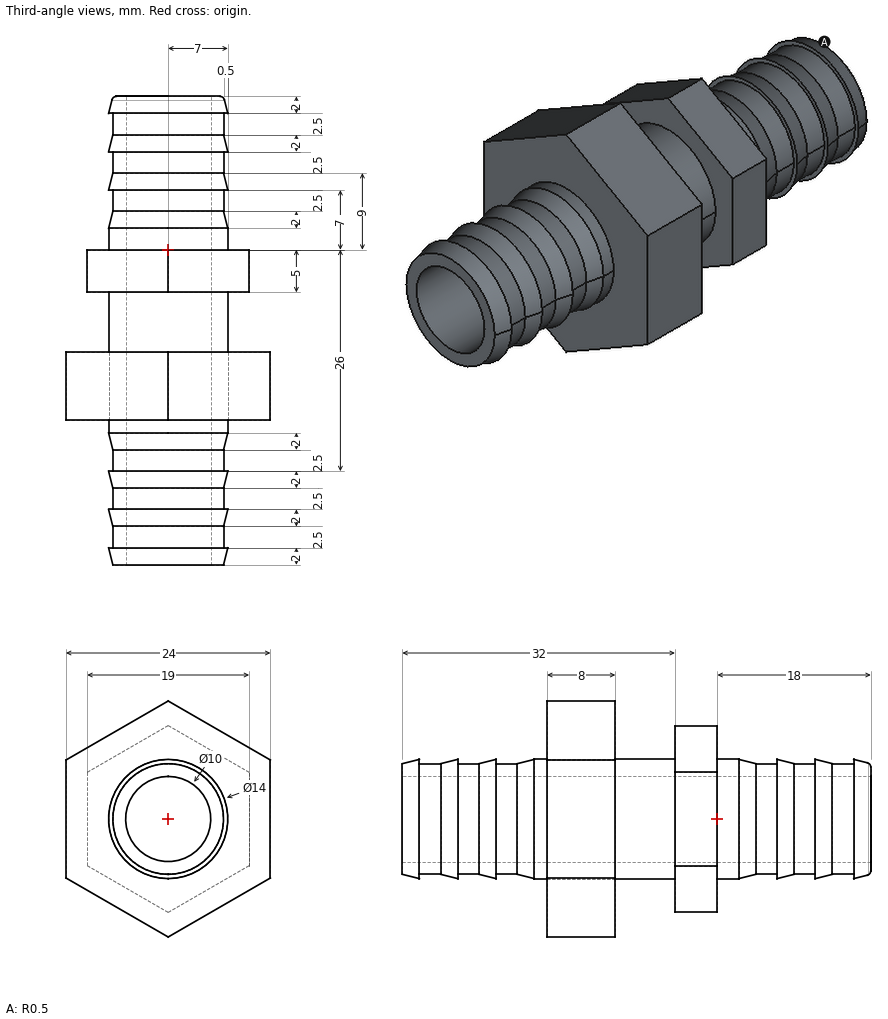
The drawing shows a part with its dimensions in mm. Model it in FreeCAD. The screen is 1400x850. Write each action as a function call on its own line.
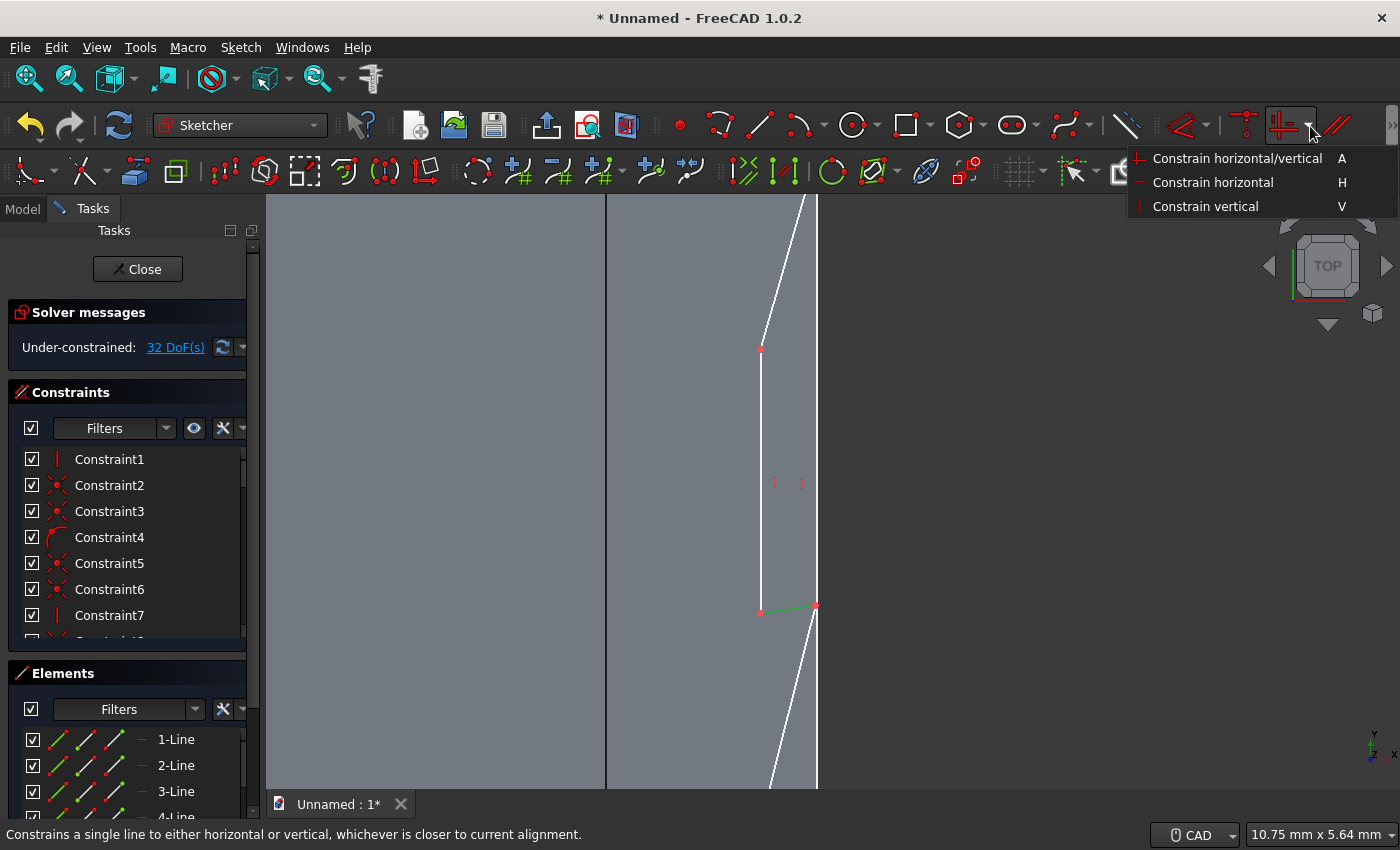
click(1263, 182)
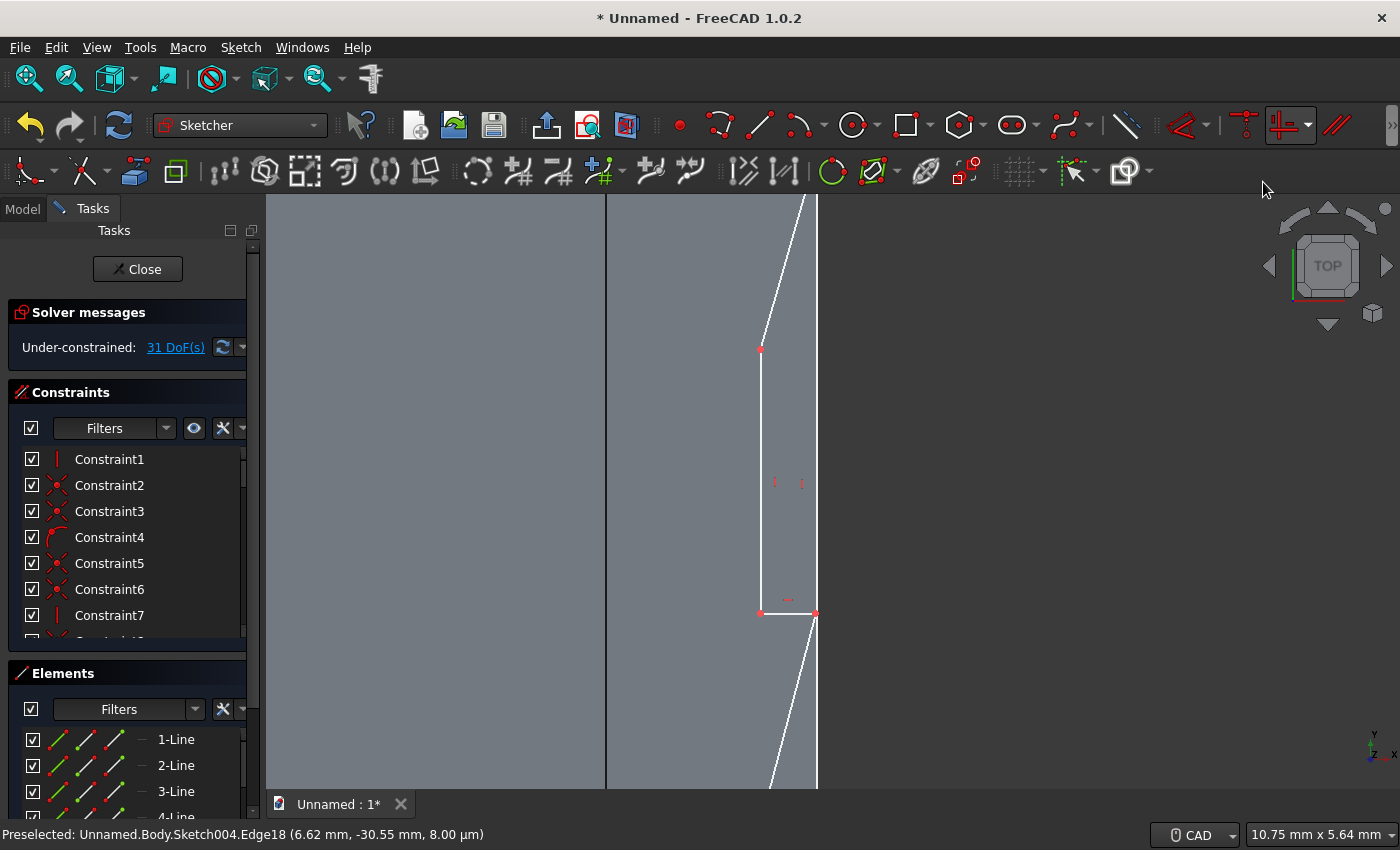
scroll(785, 627, down, 14)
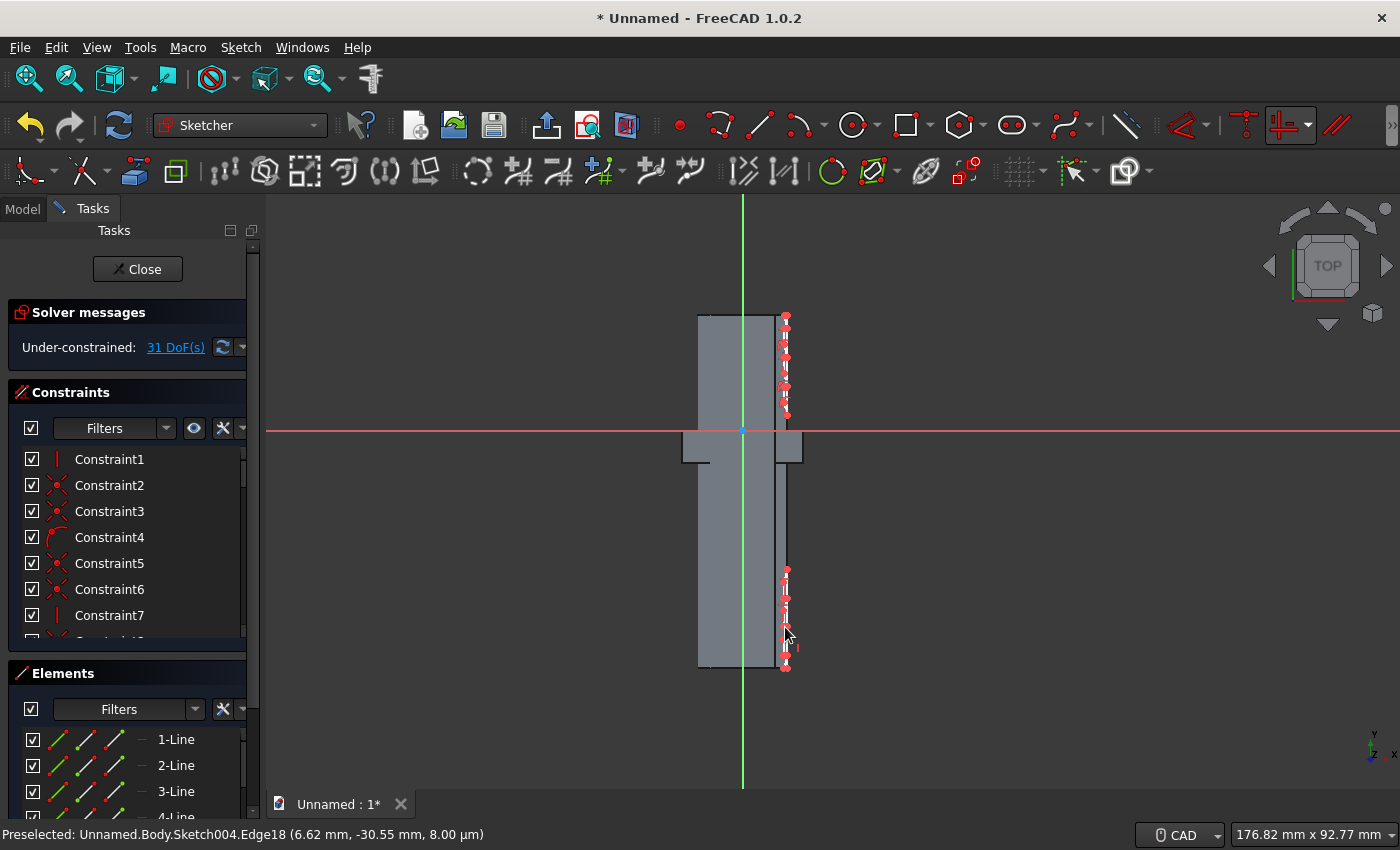
scroll(785, 656, up, 13)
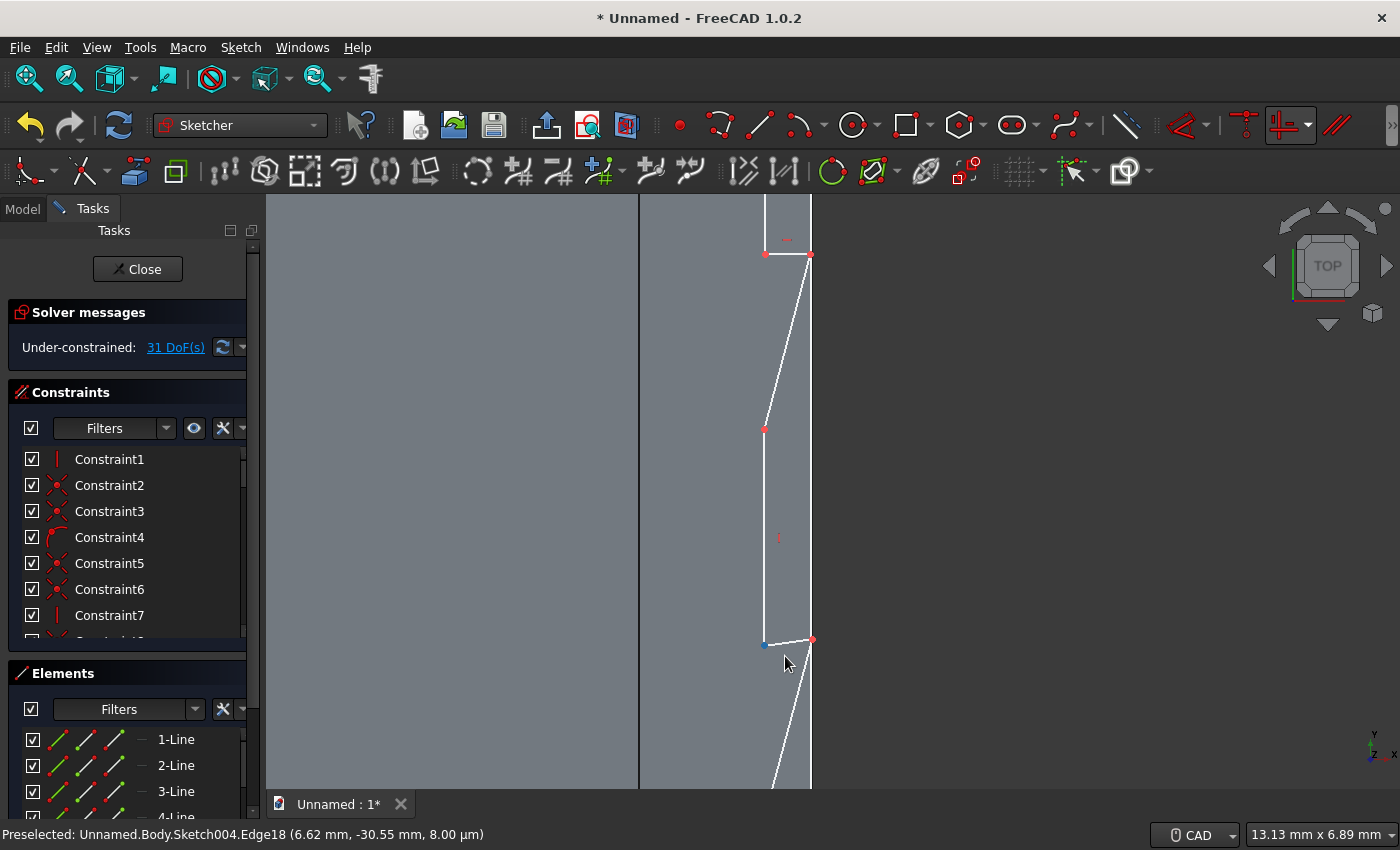
click(779, 644)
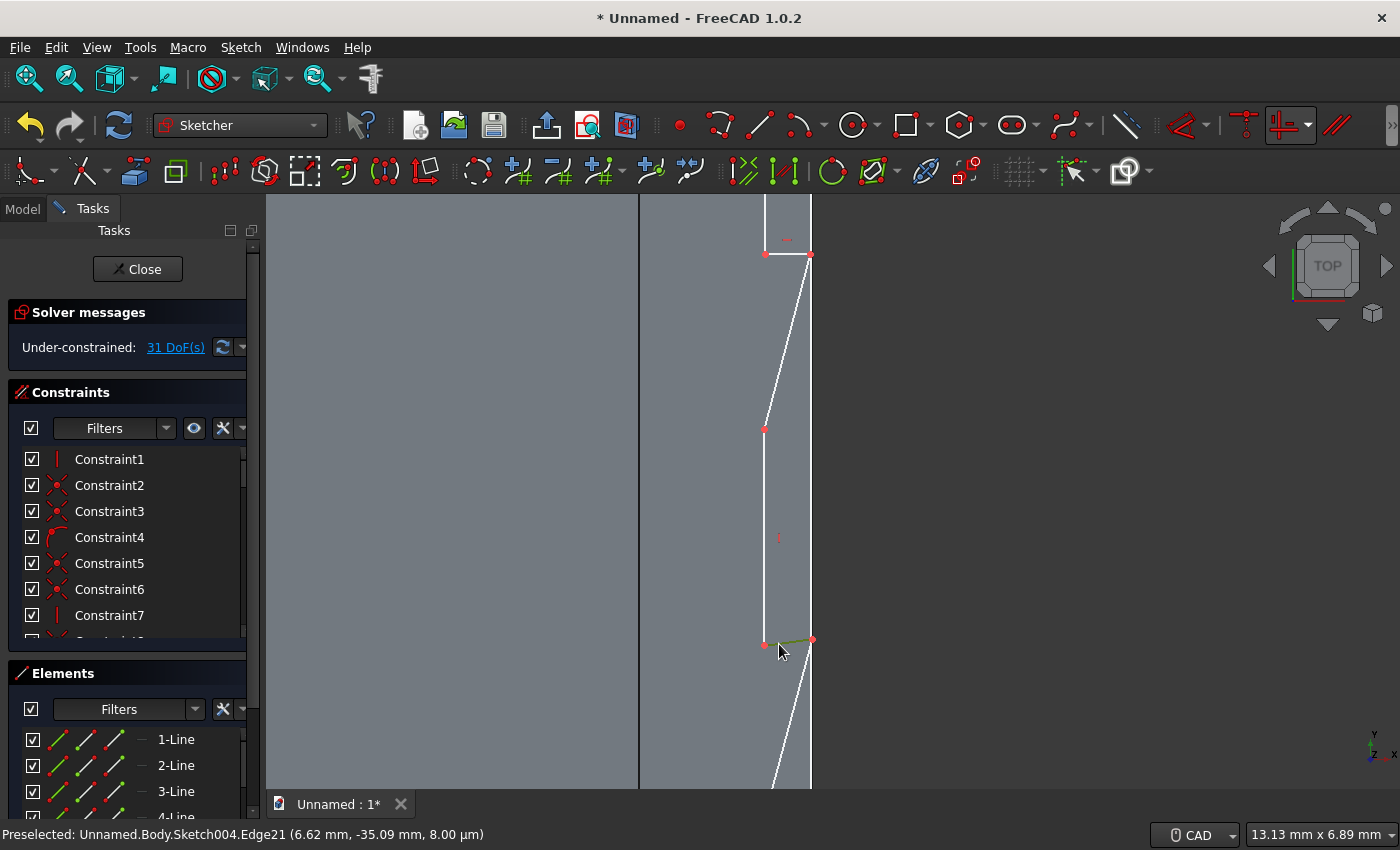
click(1310, 126)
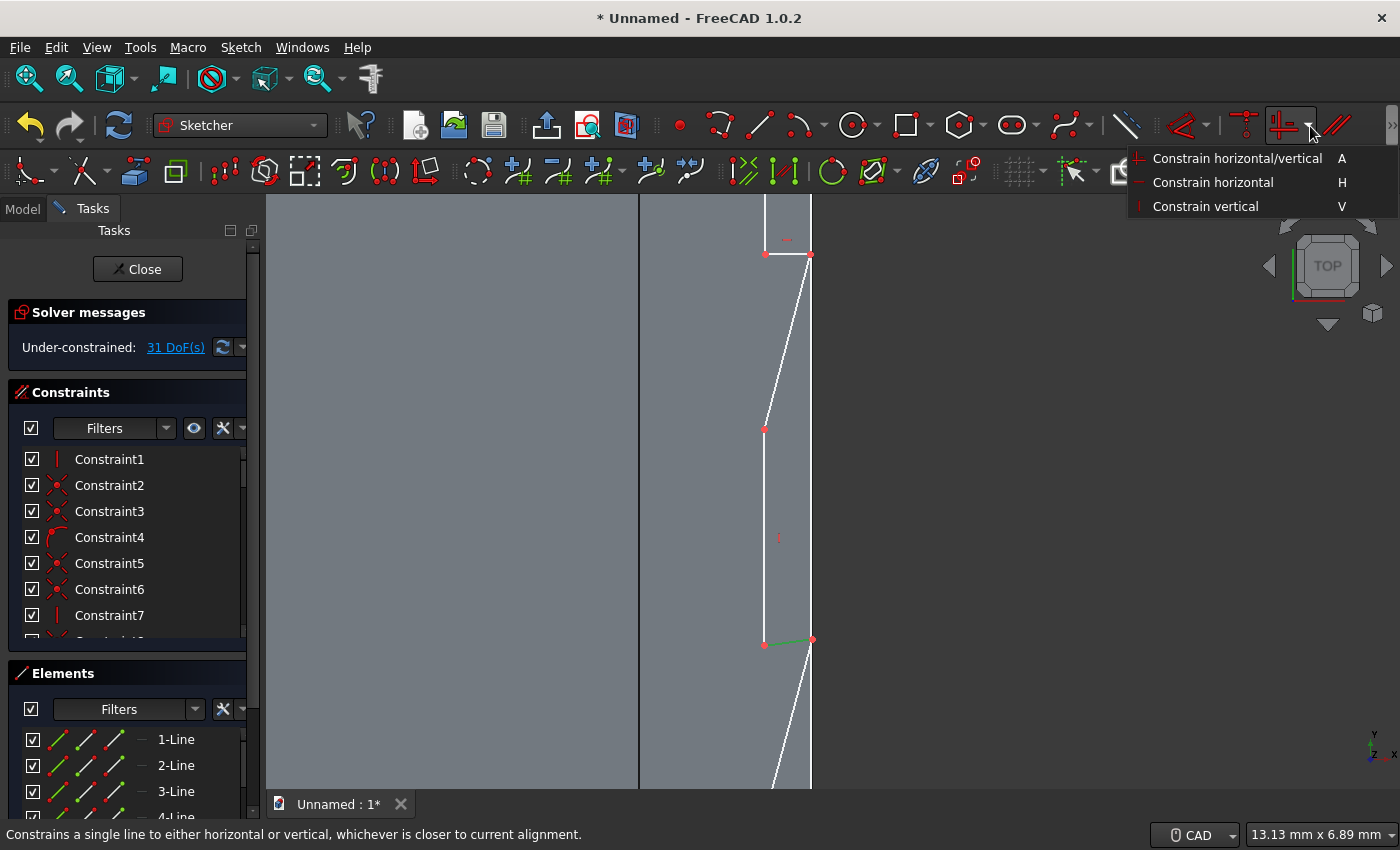
click(1263, 182)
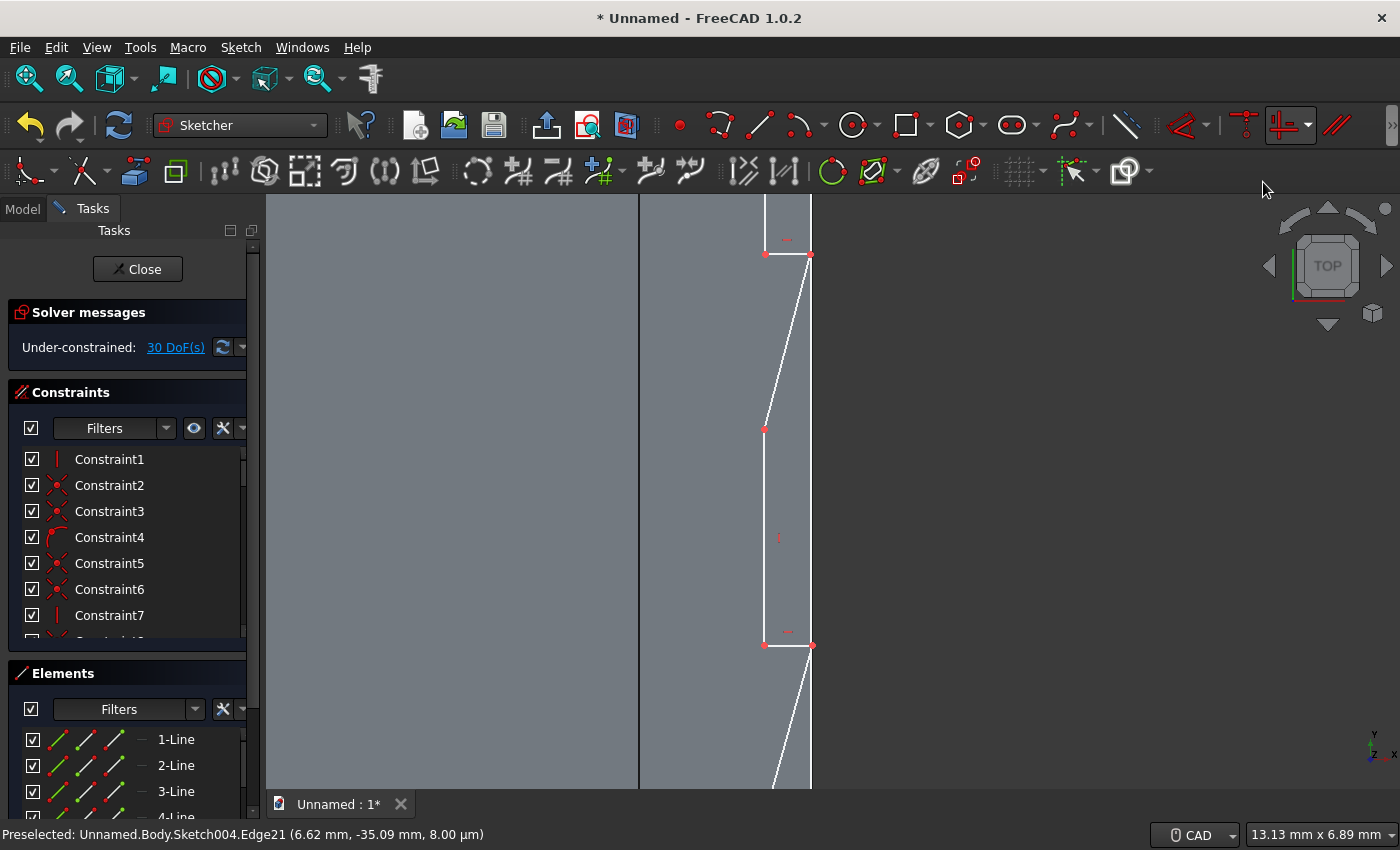
scroll(785, 657, down, 13)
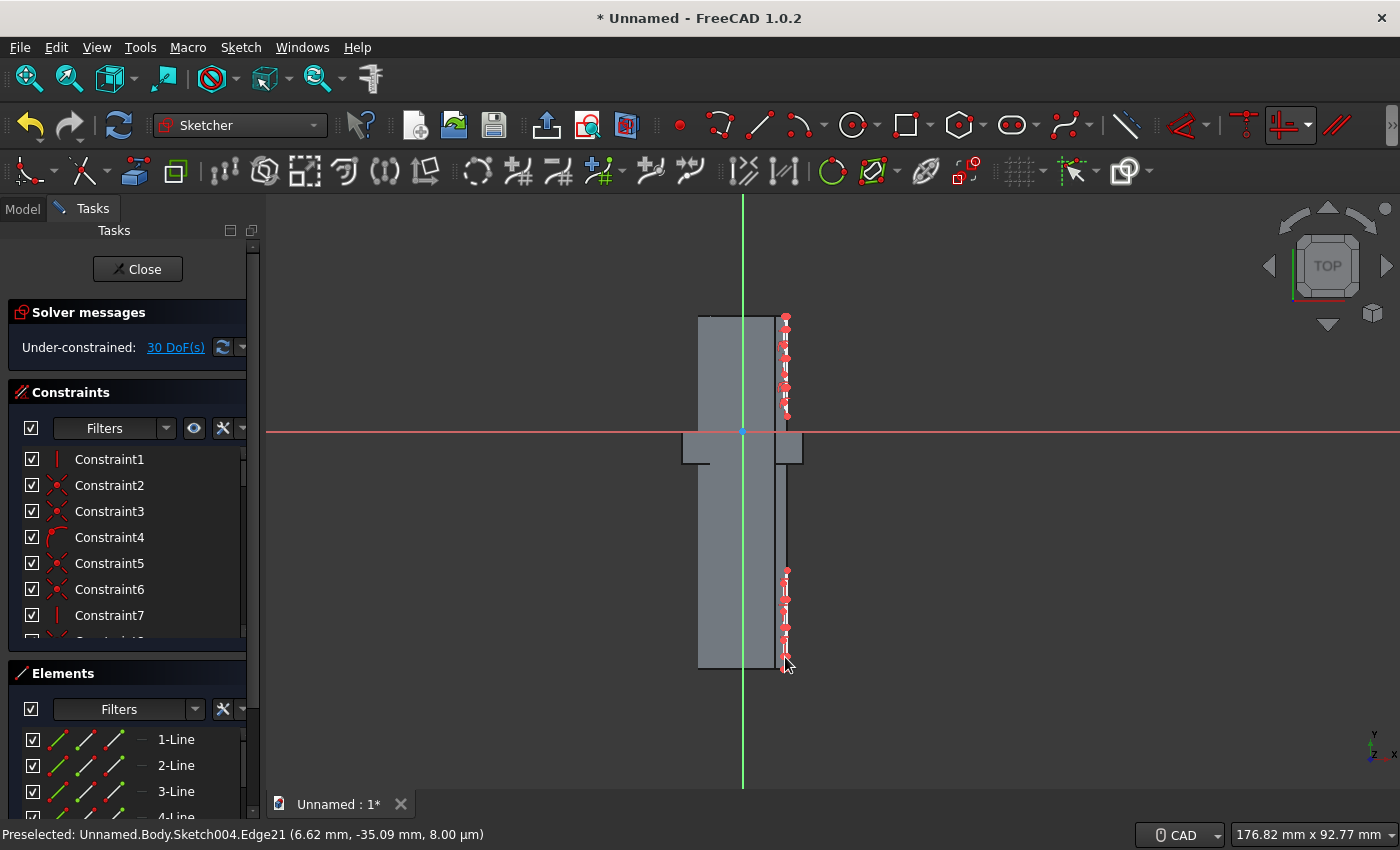
scroll(785, 669, up, 14)